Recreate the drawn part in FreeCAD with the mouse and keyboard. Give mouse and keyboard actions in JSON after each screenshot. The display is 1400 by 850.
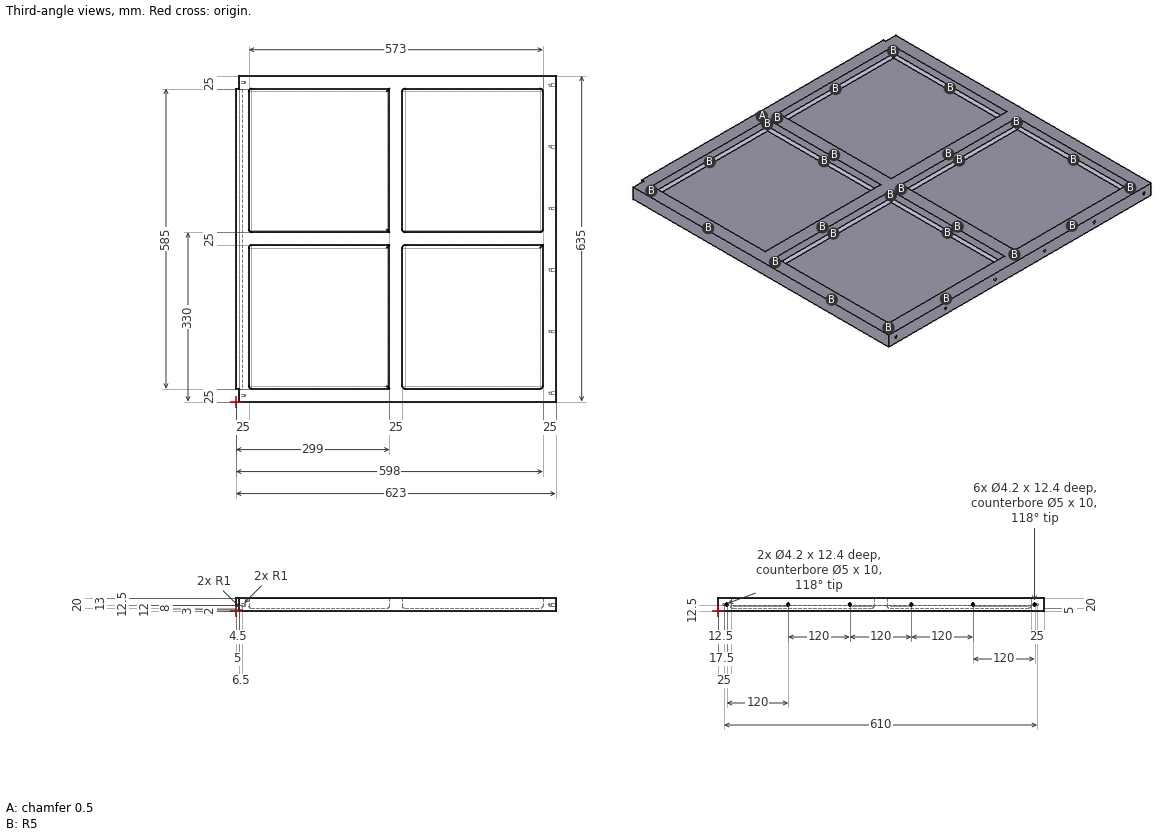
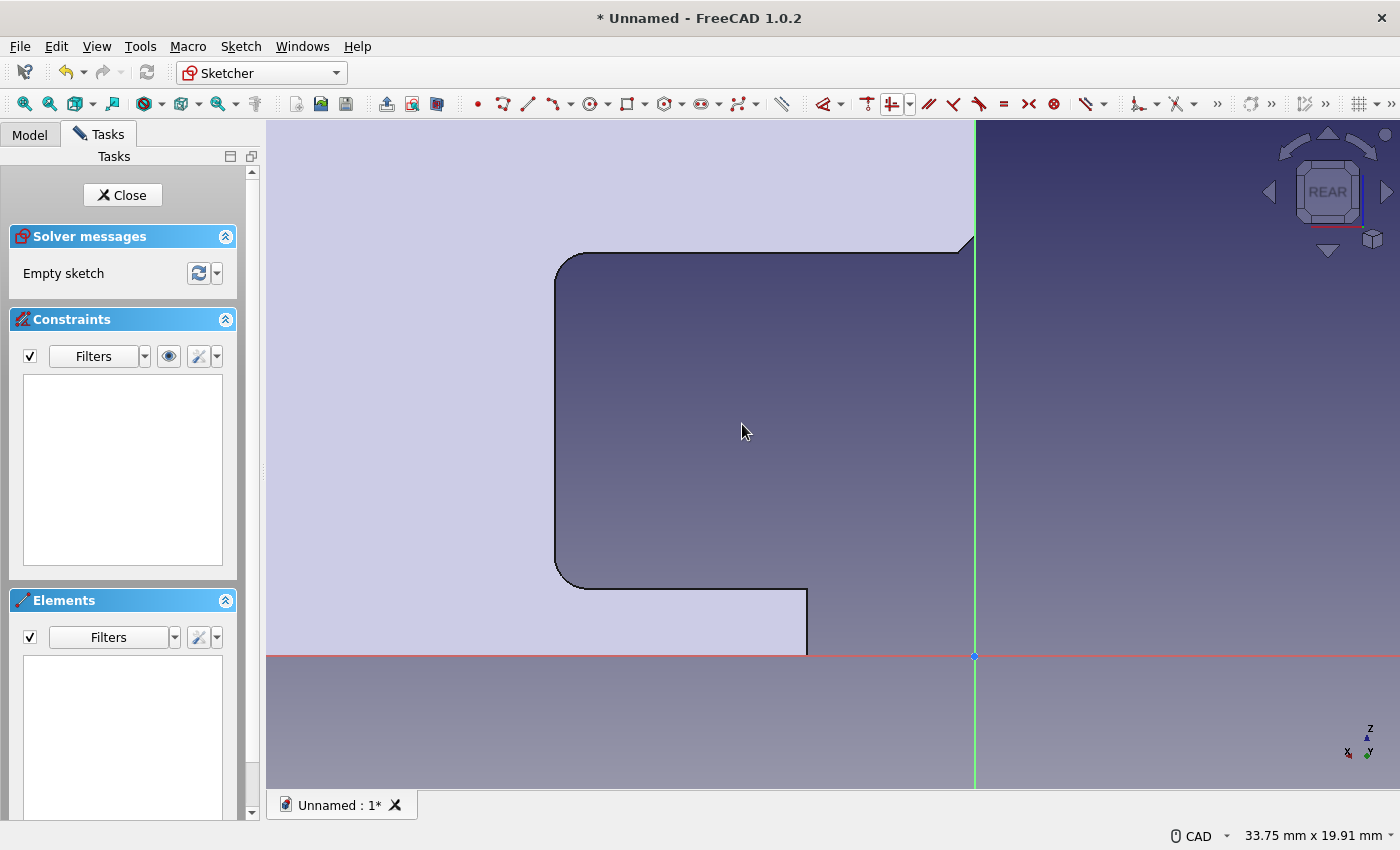
{"action": "left_click", "coordinate": [528, 104]}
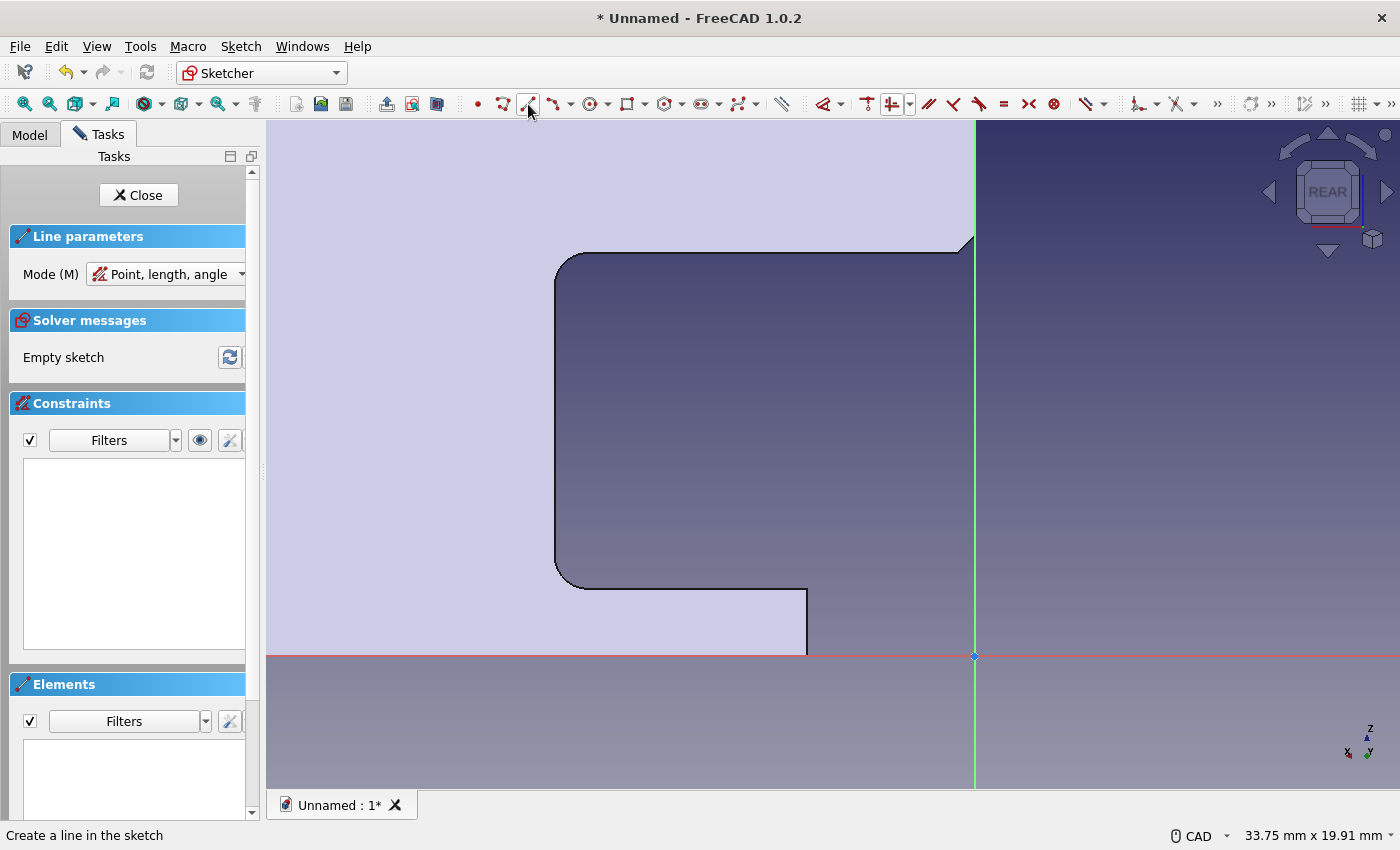
{"action": "left_click", "coordinate": [555, 286]}
{"action": "left_click", "coordinate": [555, 555]}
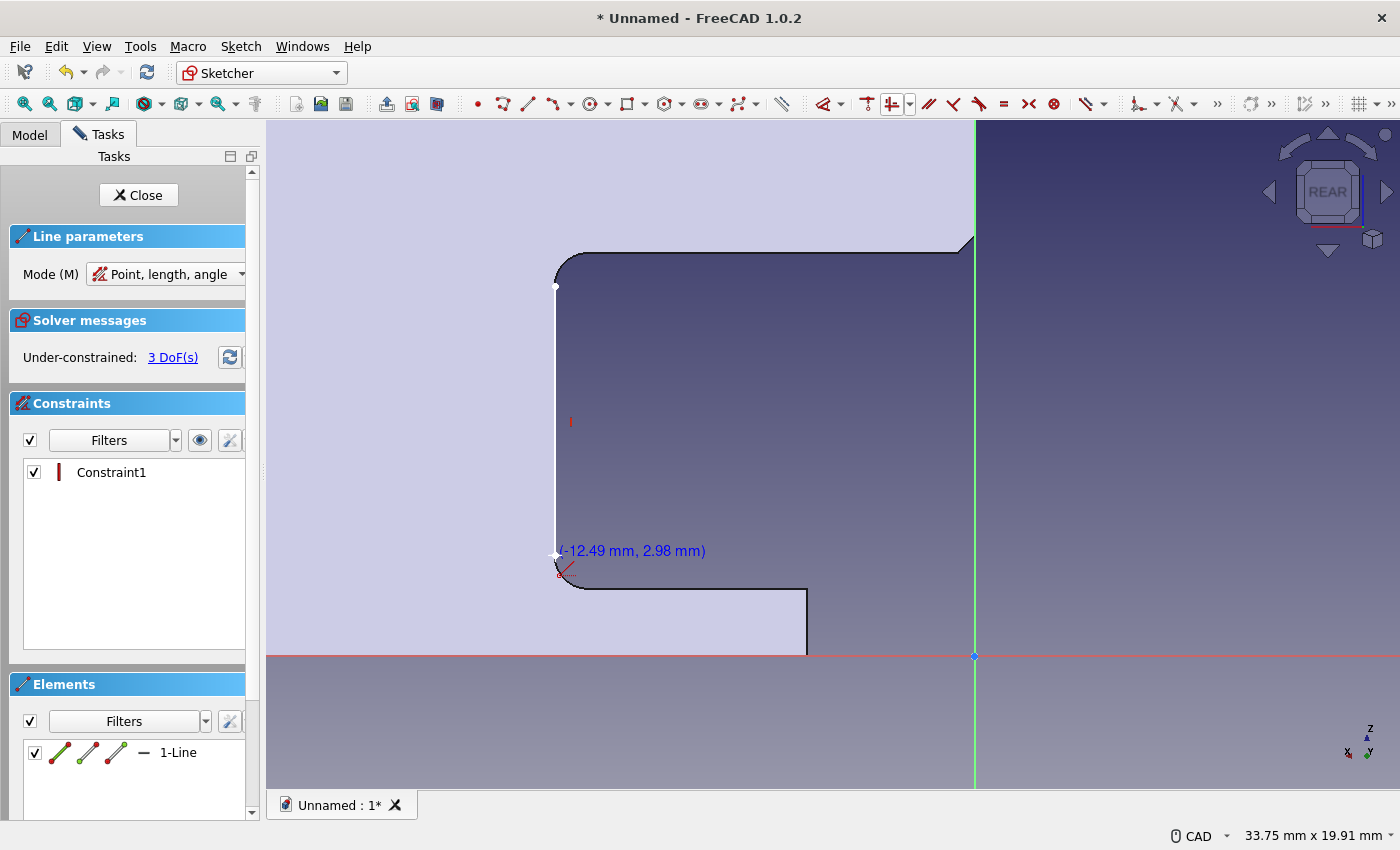
{"action": "left_click", "coordinate": [503, 104]}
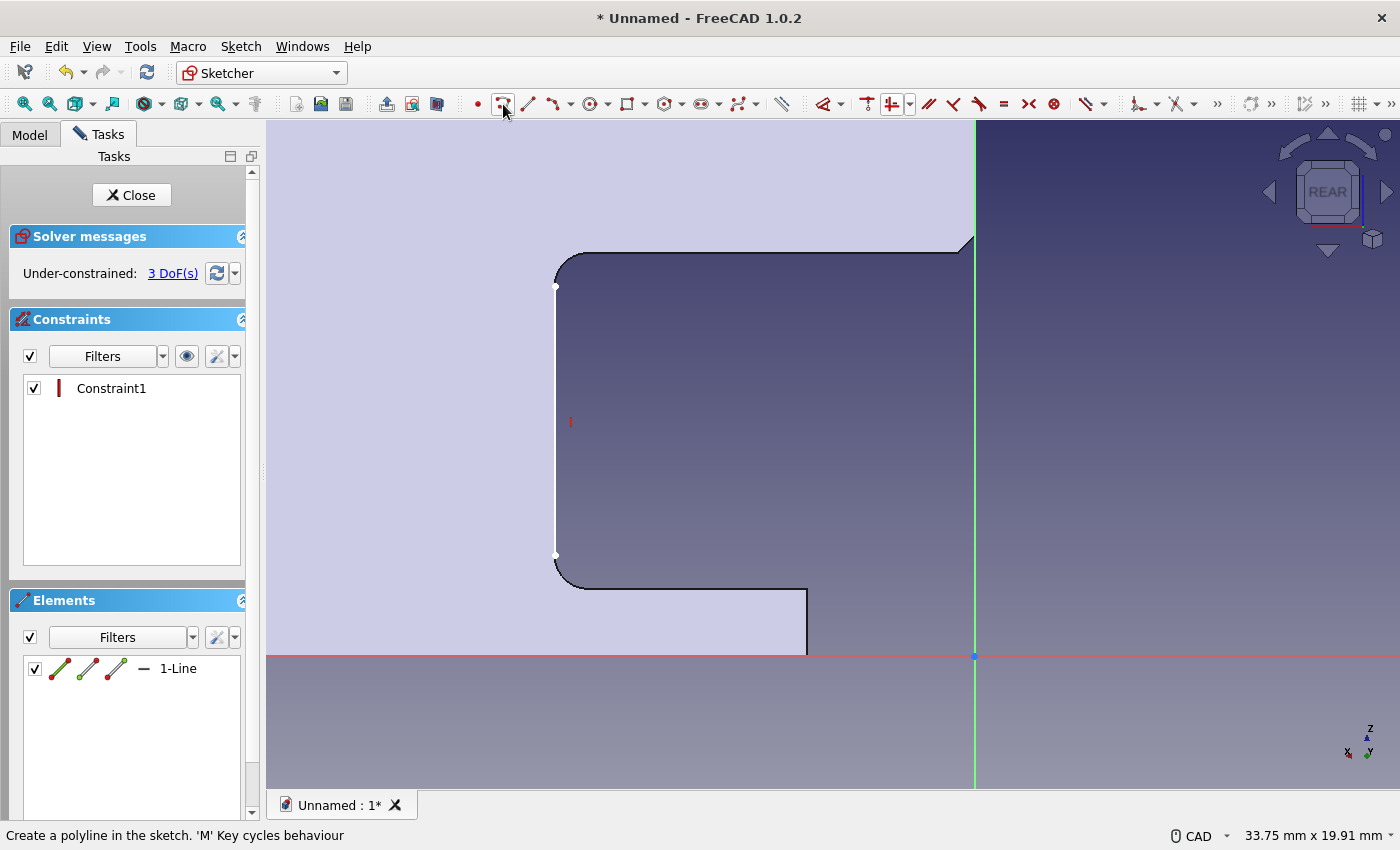
{"action": "left_click", "coordinate": [588, 589]}
{"action": "left_click", "coordinate": [807, 589]}
{"action": "left_click", "coordinate": [807, 253]}
{"action": "left_click", "coordinate": [588, 253]}
{"action": "right_click", "coordinate": [588, 253]}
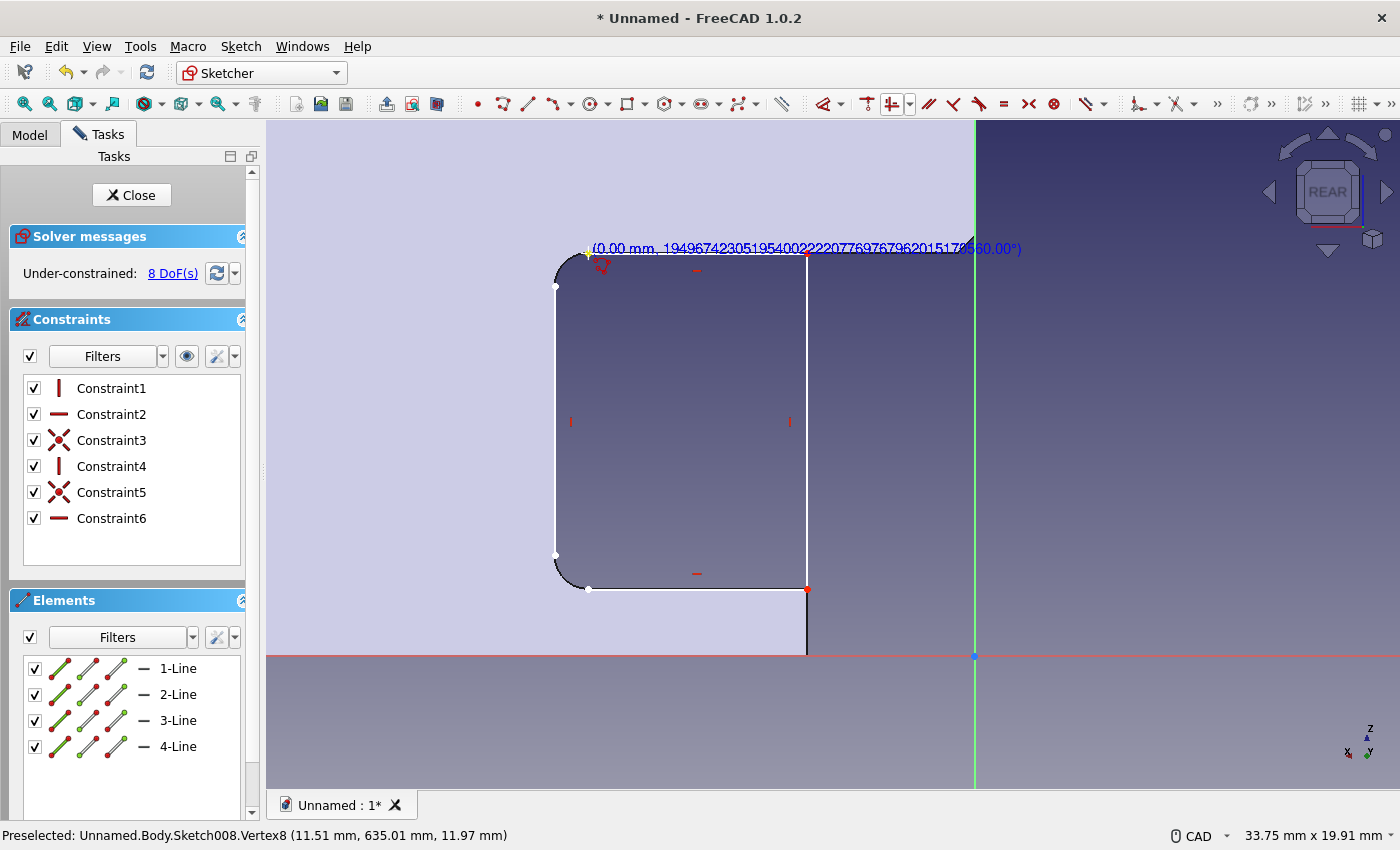
{"action": "left_click", "coordinate": [552, 104]}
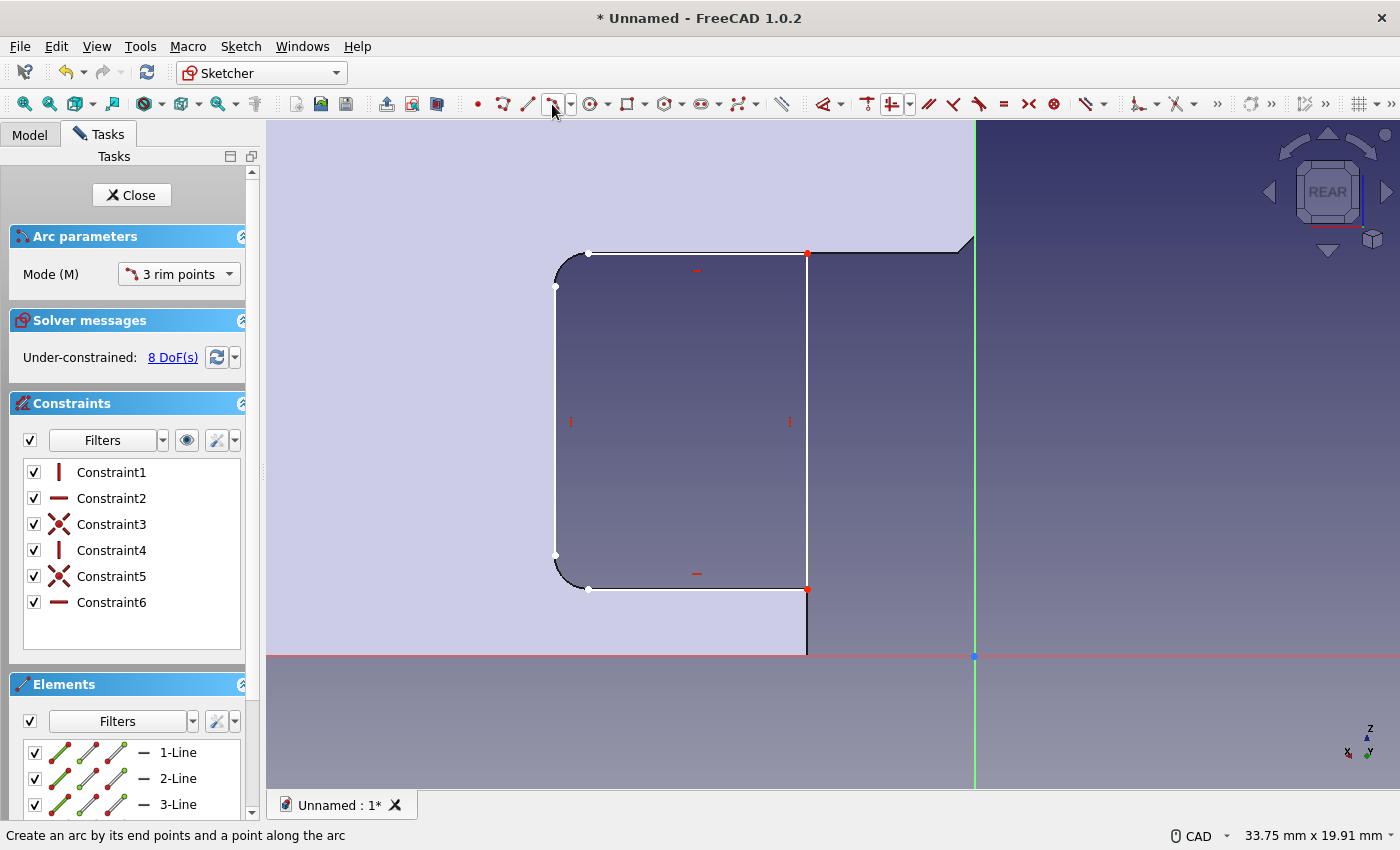
{"action": "left_click", "coordinate": [555, 556]}
{"action": "left_click", "coordinate": [588, 590]}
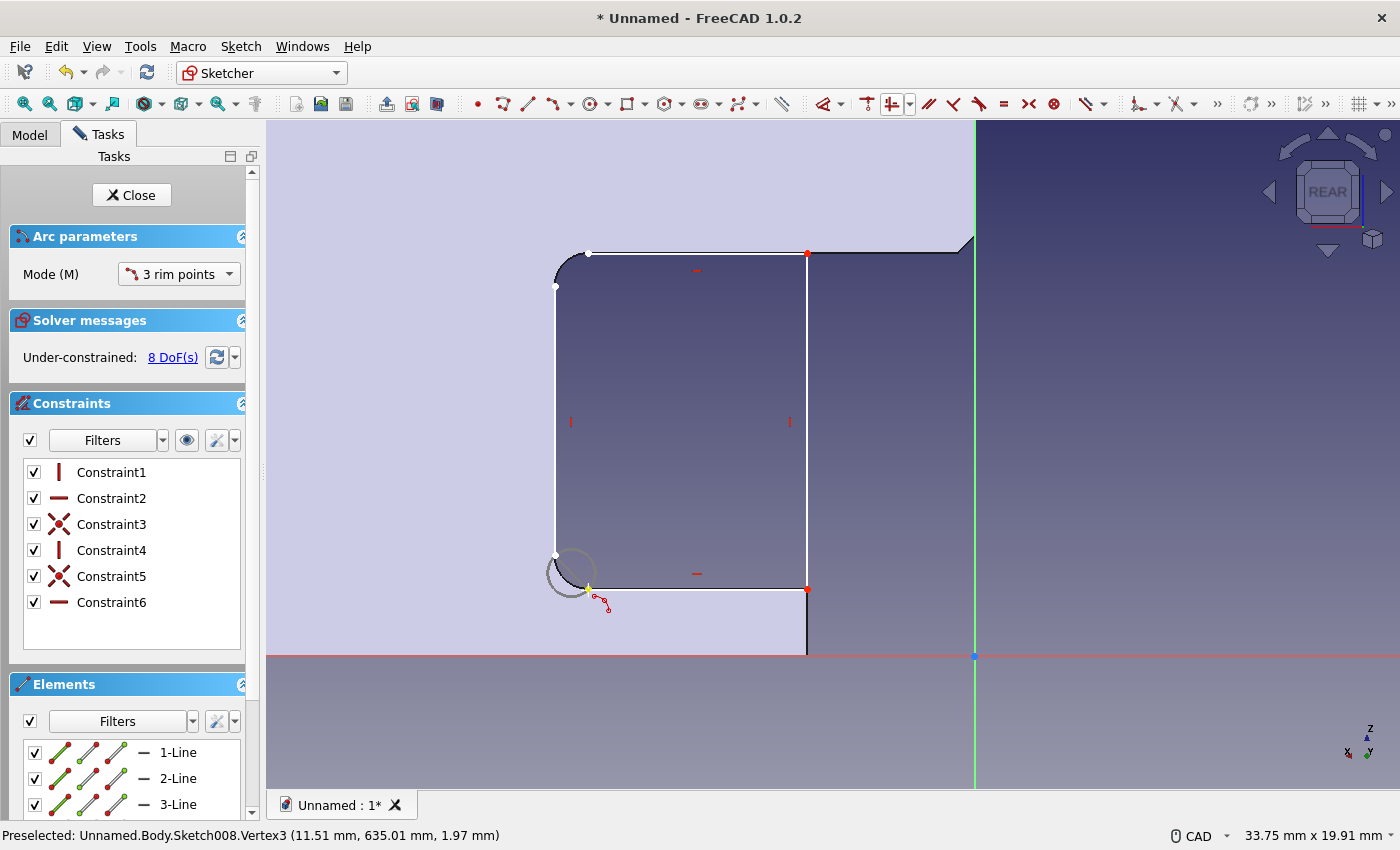
{"action": "scroll", "coordinate": [564, 579], "scroll_direction": "up", "scroll_amount": 3}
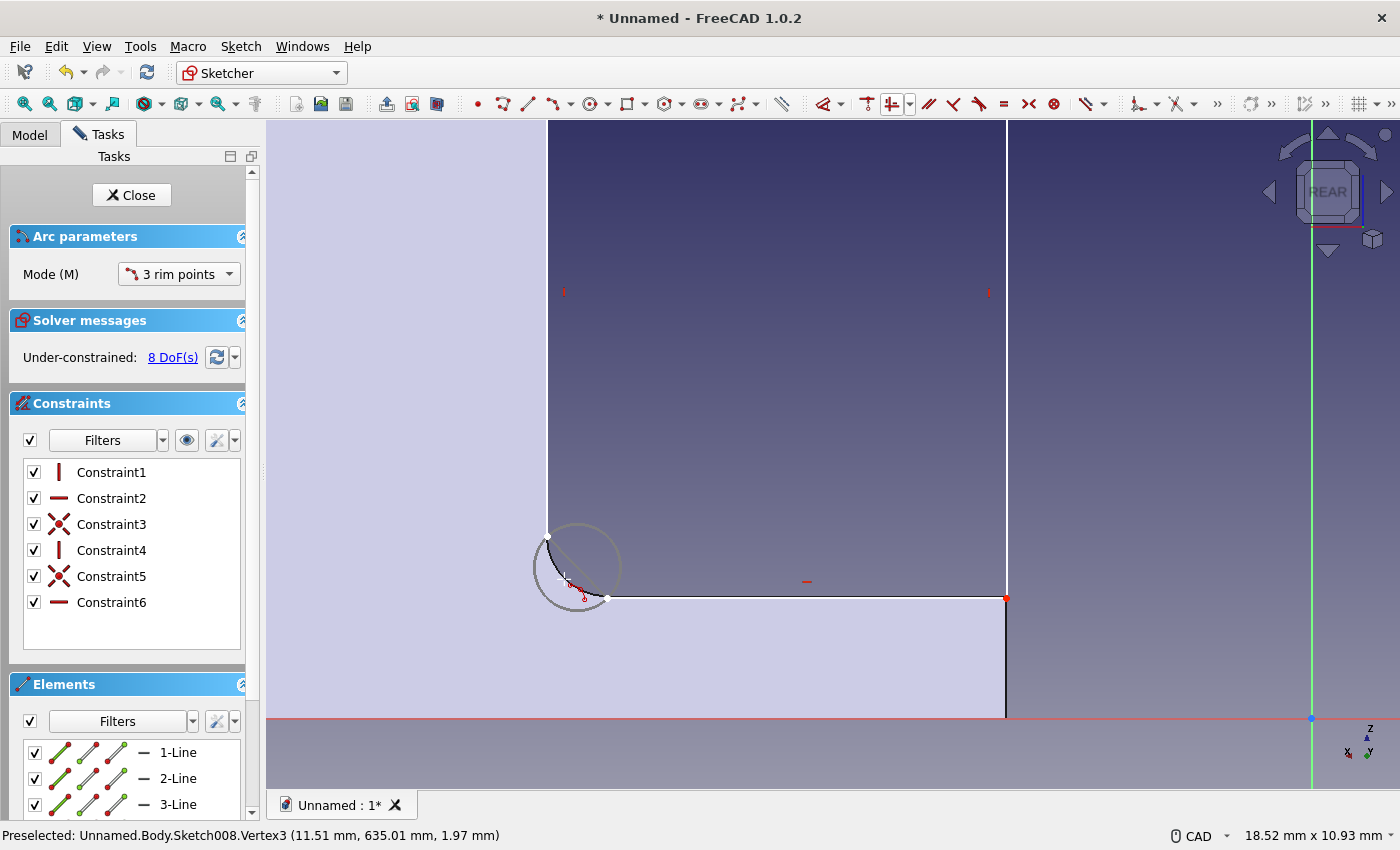
{"action": "left_click", "coordinate": [565, 579]}